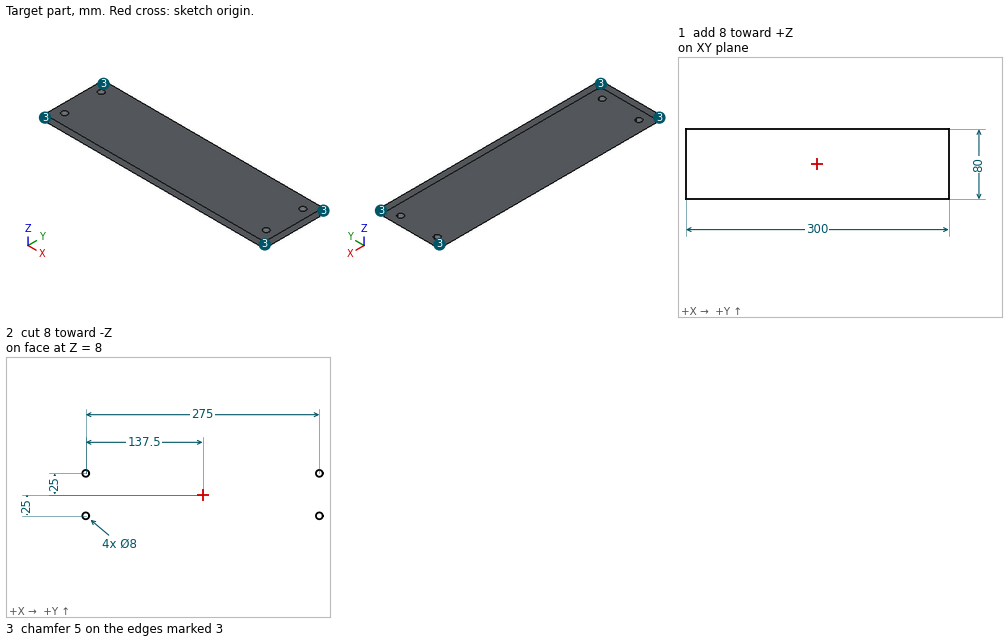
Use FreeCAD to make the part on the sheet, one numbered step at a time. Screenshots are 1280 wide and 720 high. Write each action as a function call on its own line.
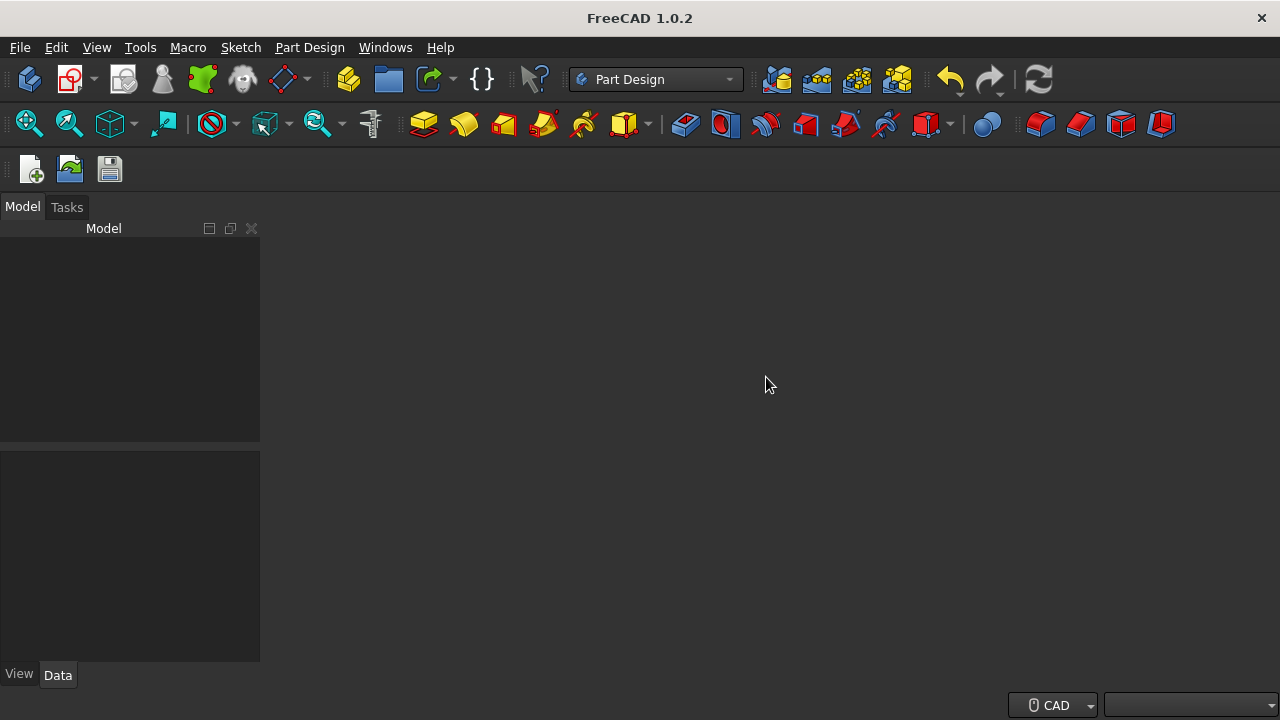
key(ctrl+n)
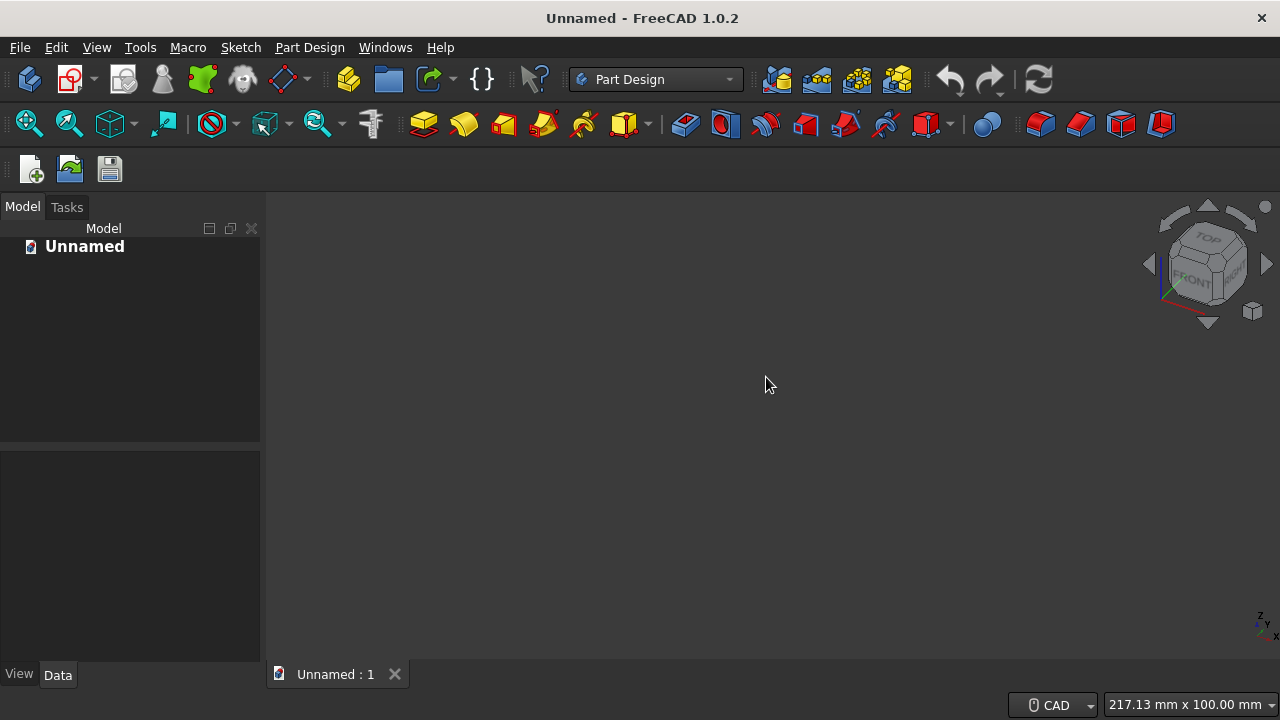
click(70, 80)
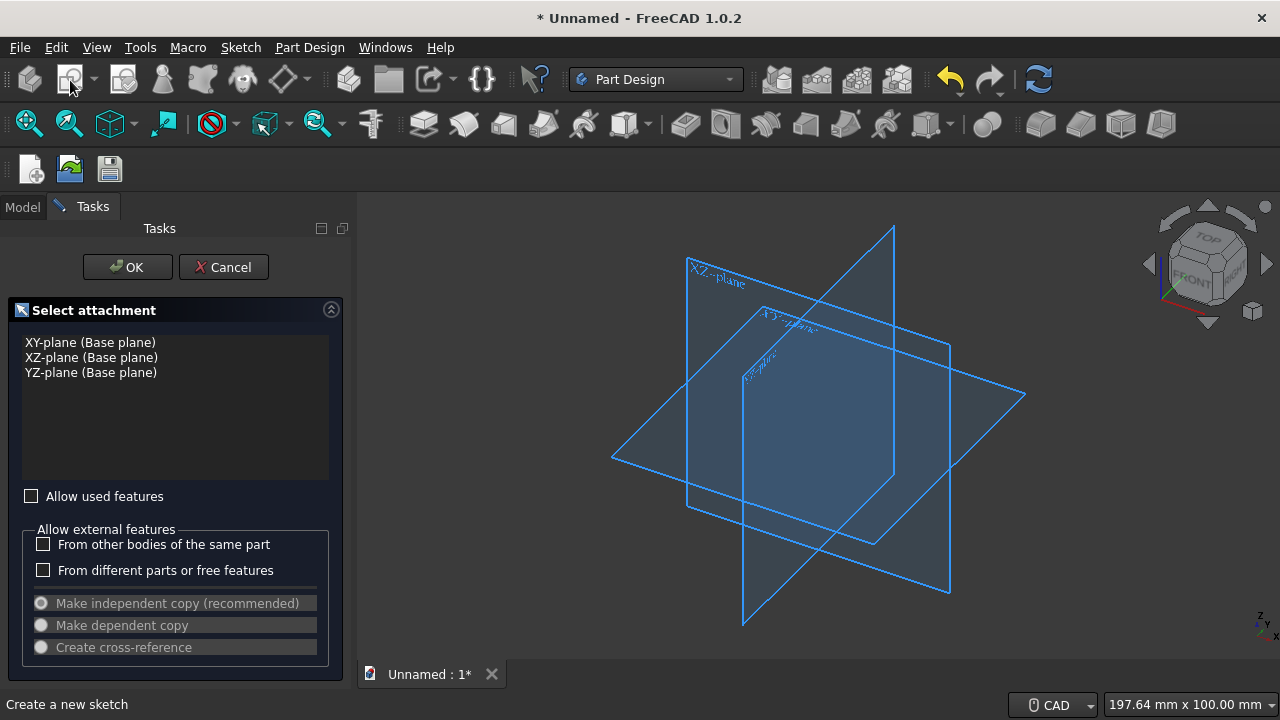
click(82, 342)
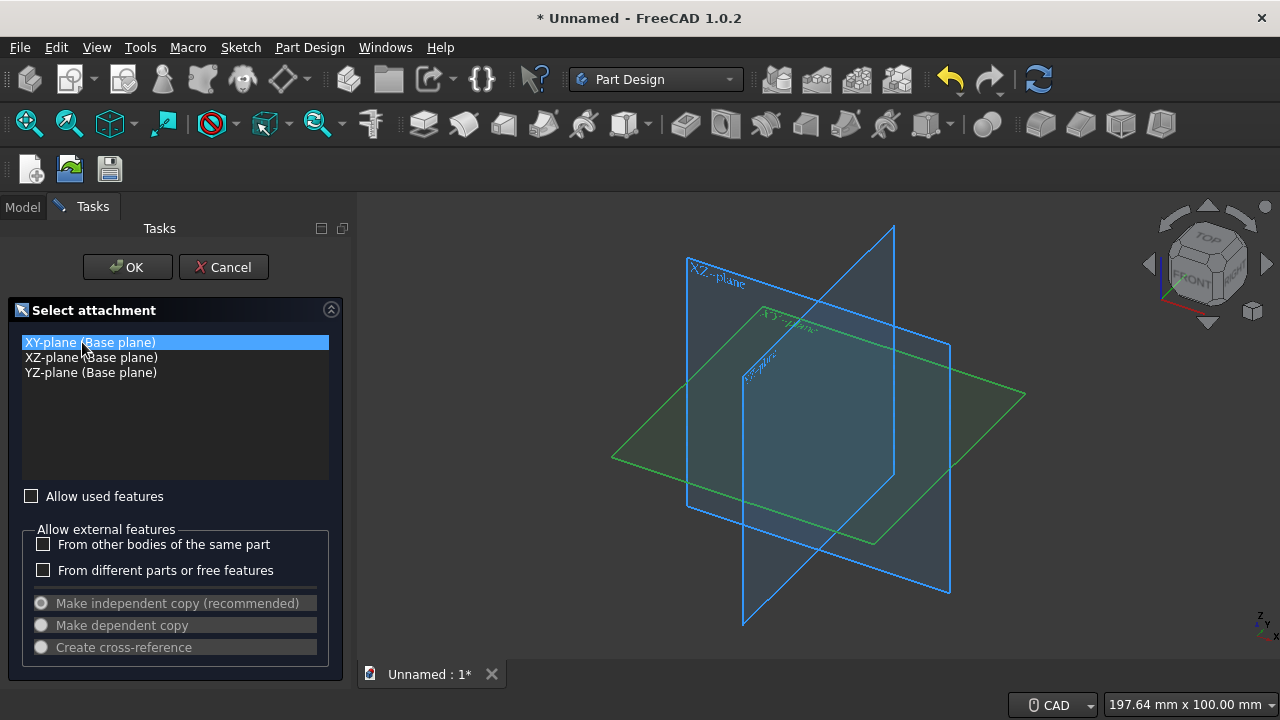
click(128, 267)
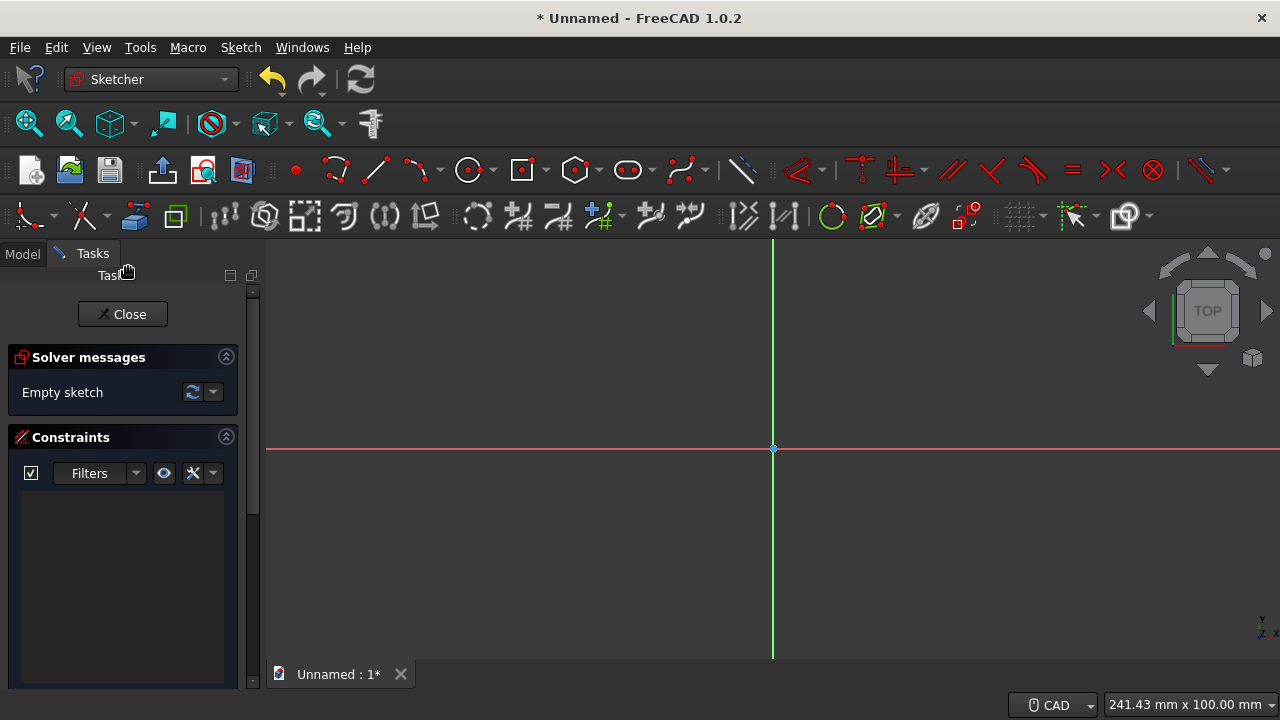
scroll(649, 449, down, 4)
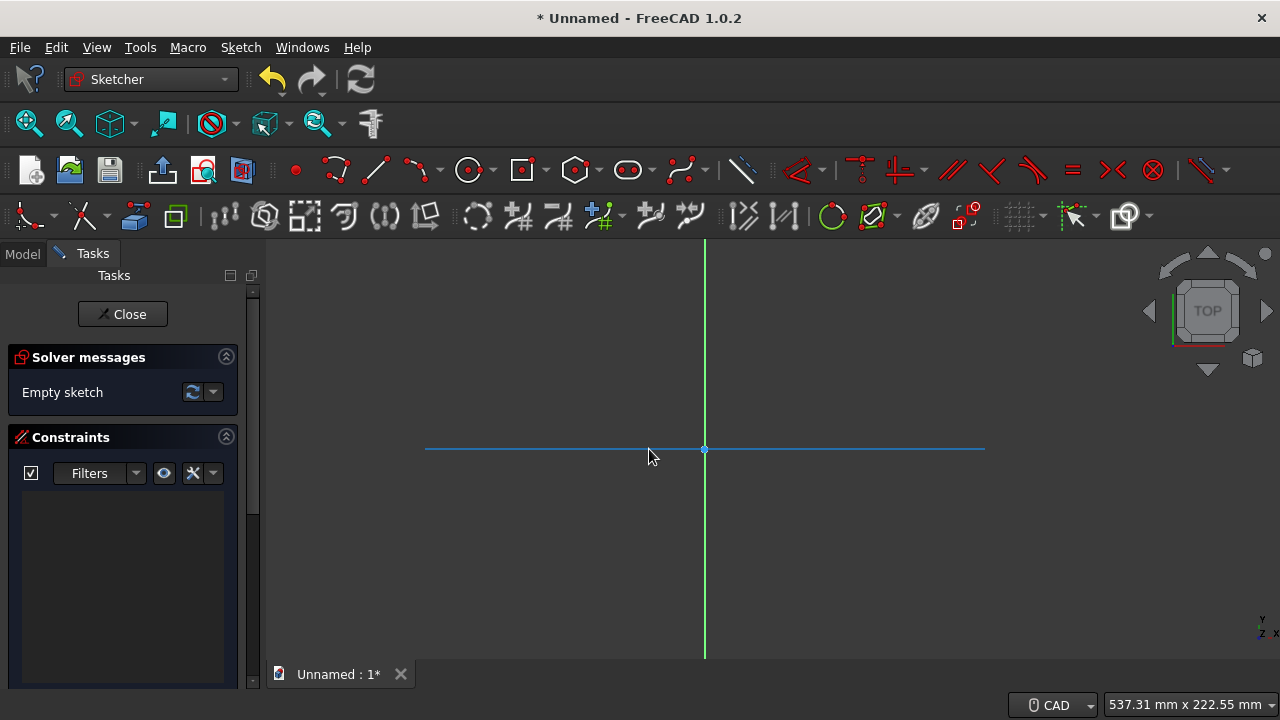
key(g)
key(v)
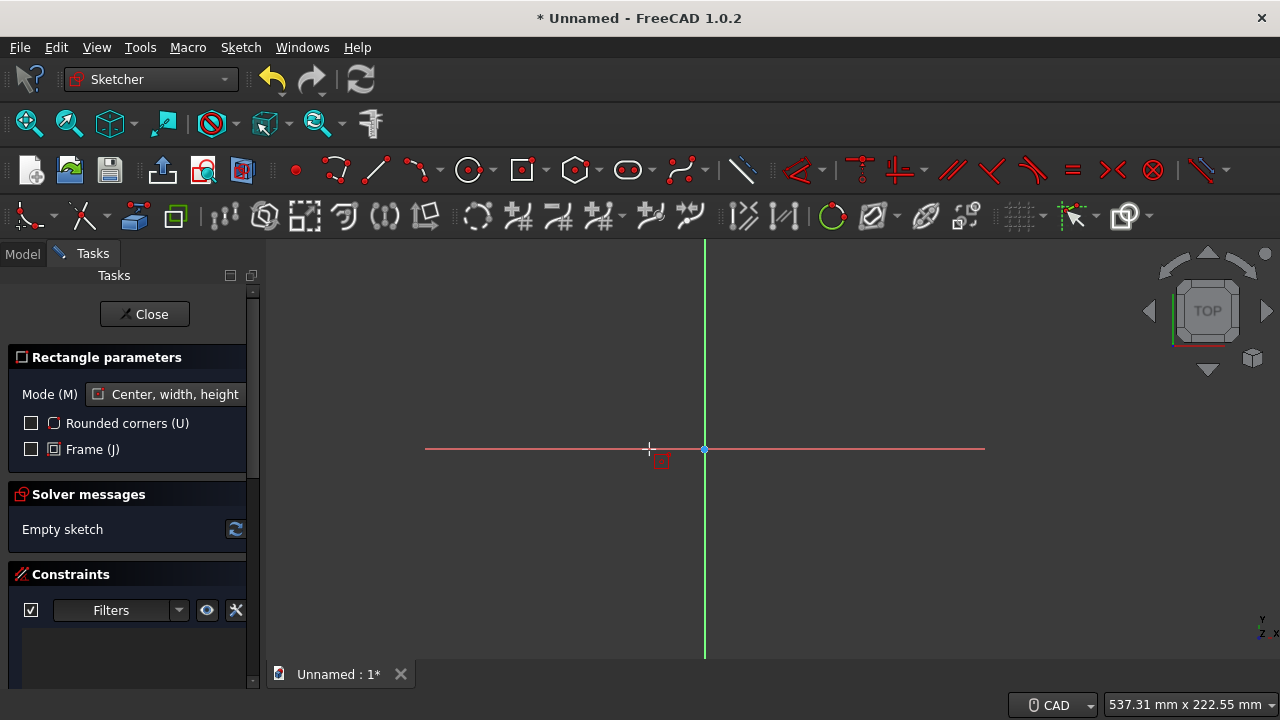
click(705, 449)
move(988, 374)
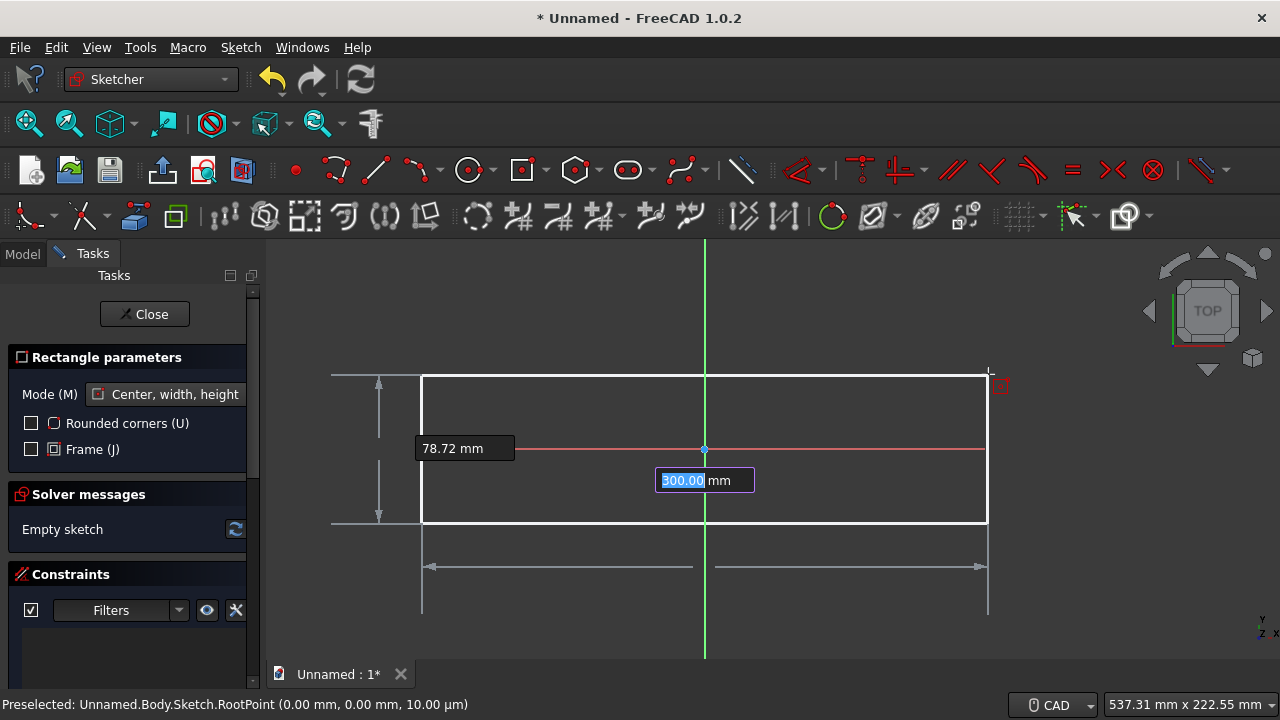
text(300)
key(Tab)
text(80)
key(Return)
key(Escape)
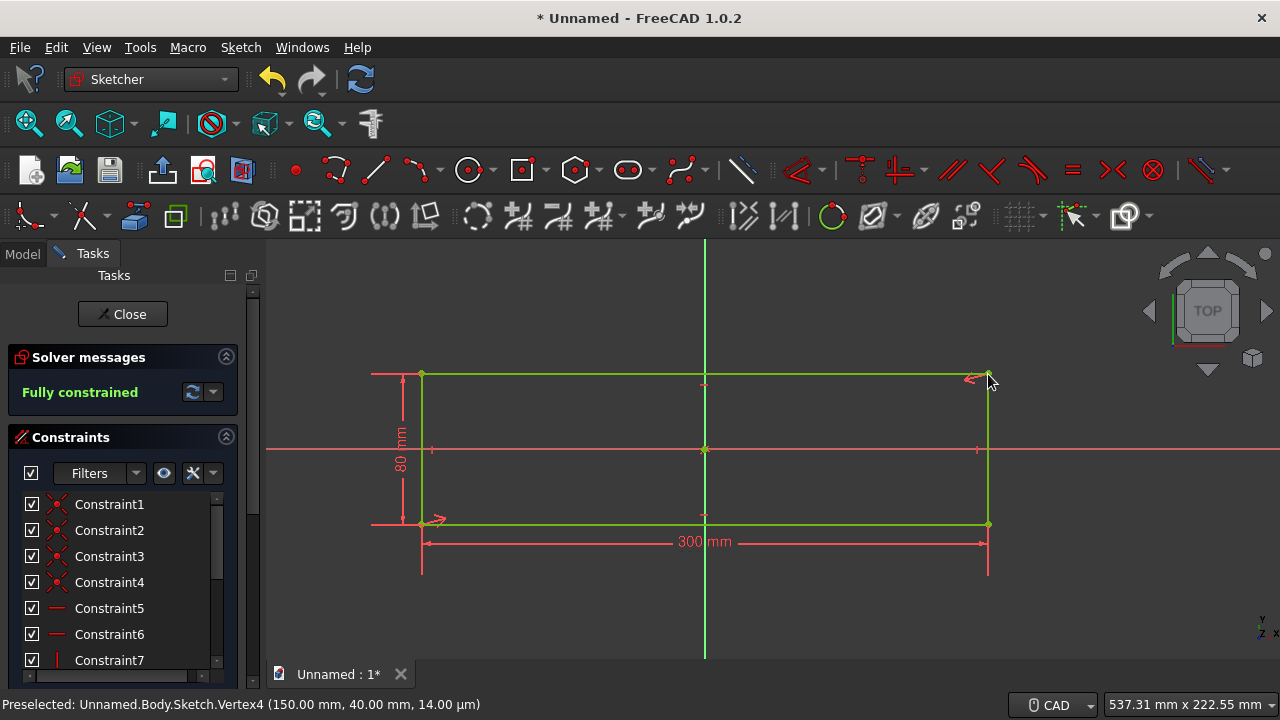
click(123, 314)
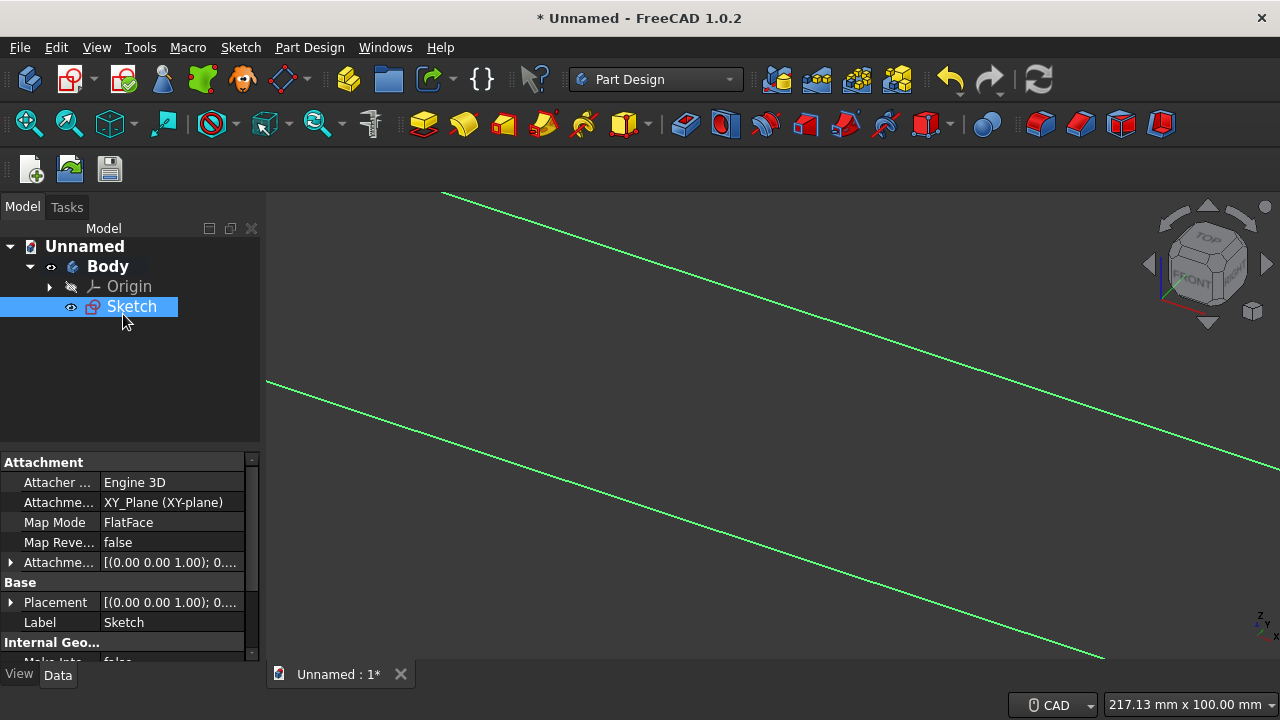
click(424, 124)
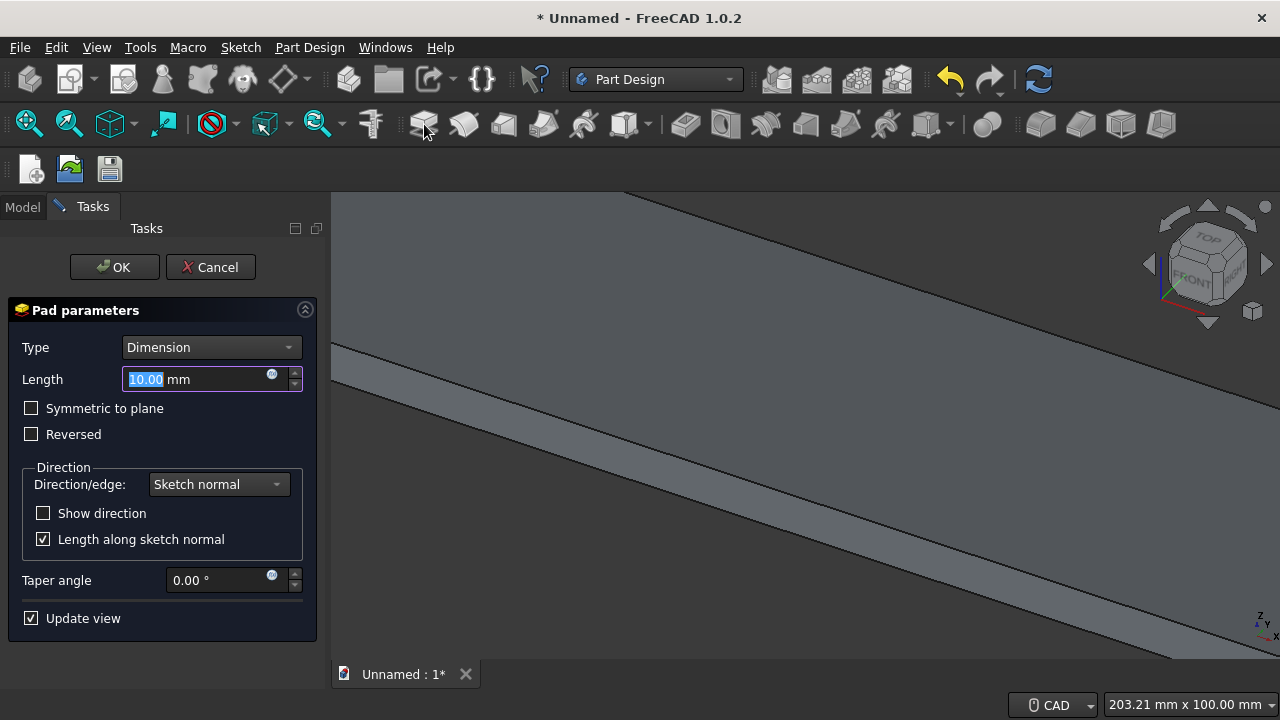
text(8)
key(Tab)